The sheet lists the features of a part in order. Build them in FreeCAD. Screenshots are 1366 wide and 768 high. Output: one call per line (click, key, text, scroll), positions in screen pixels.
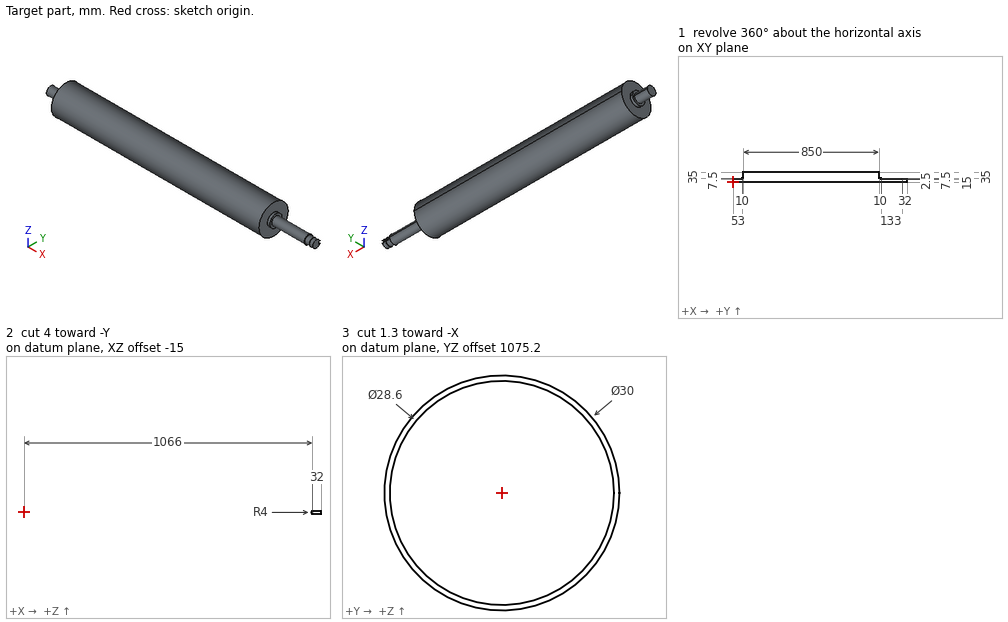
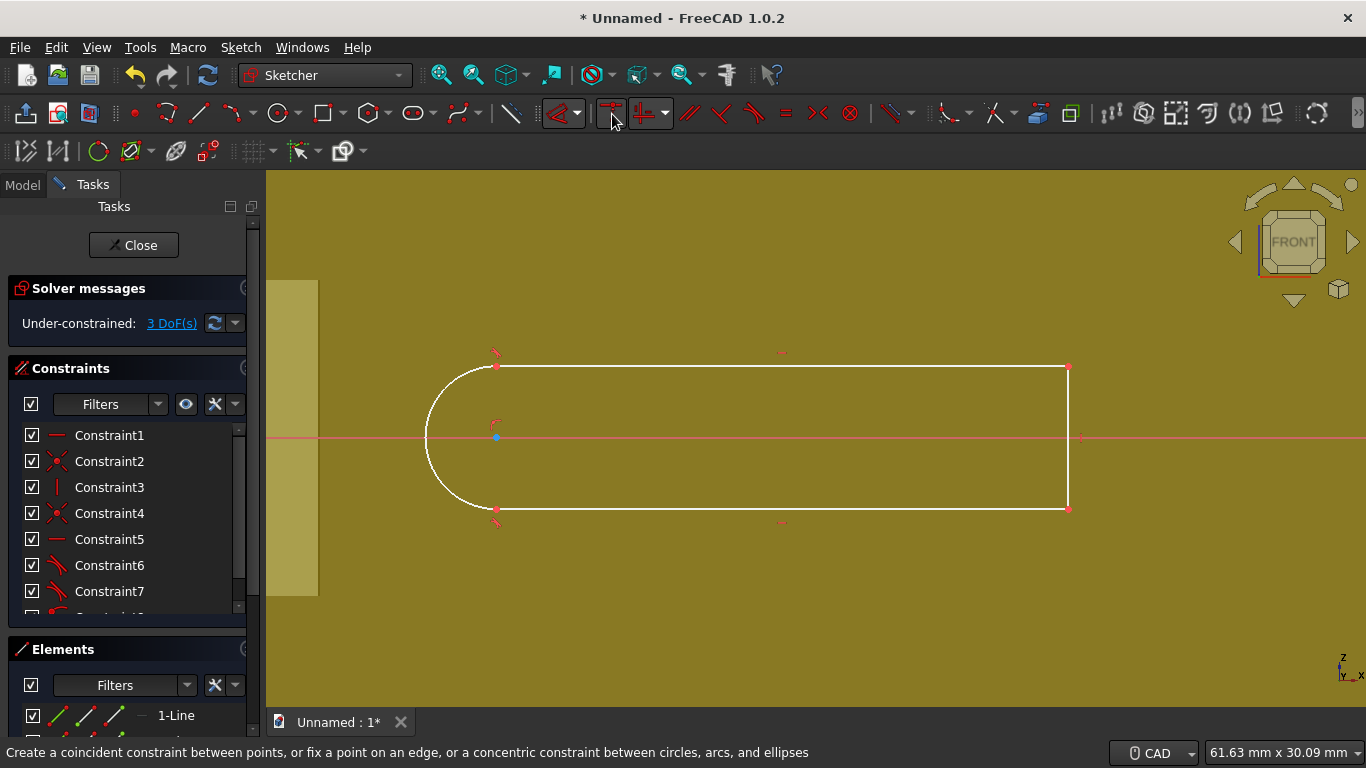
click(439, 396)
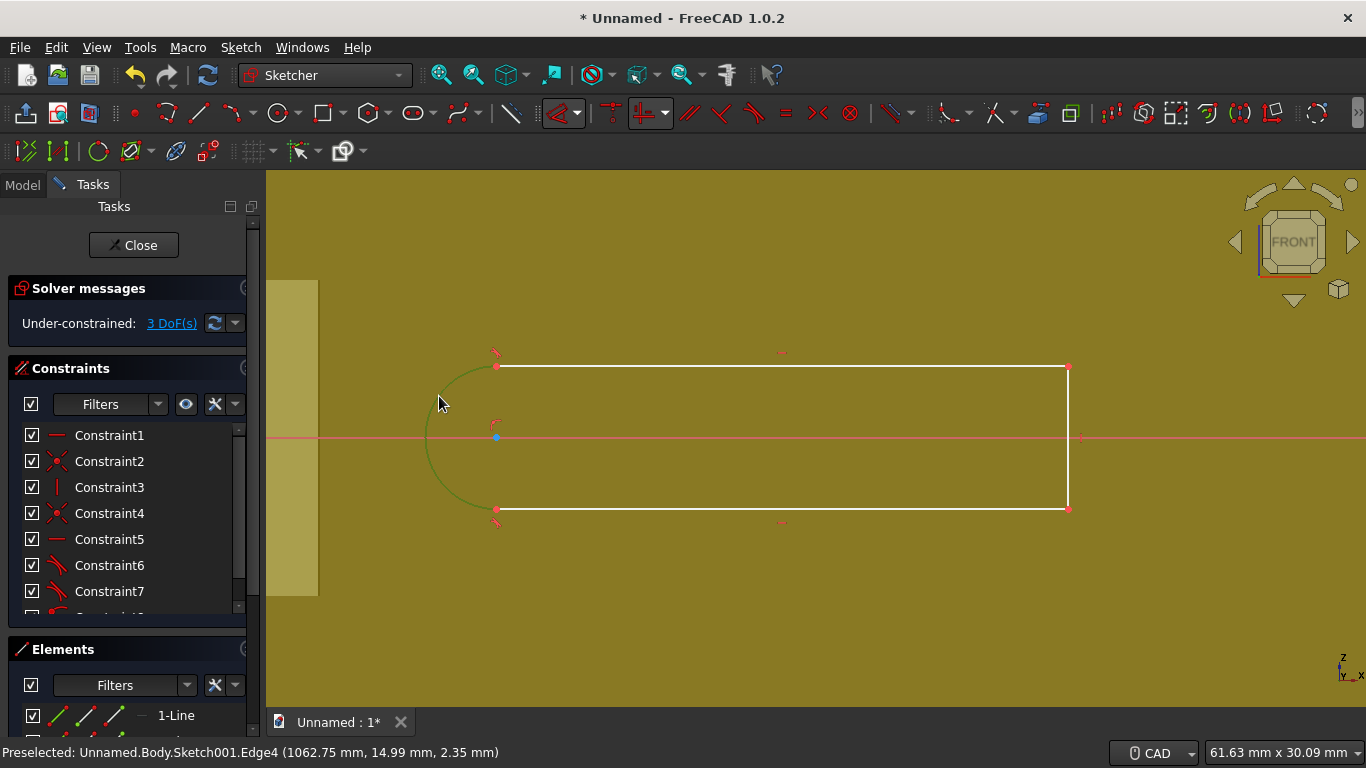
key(k)
key(r)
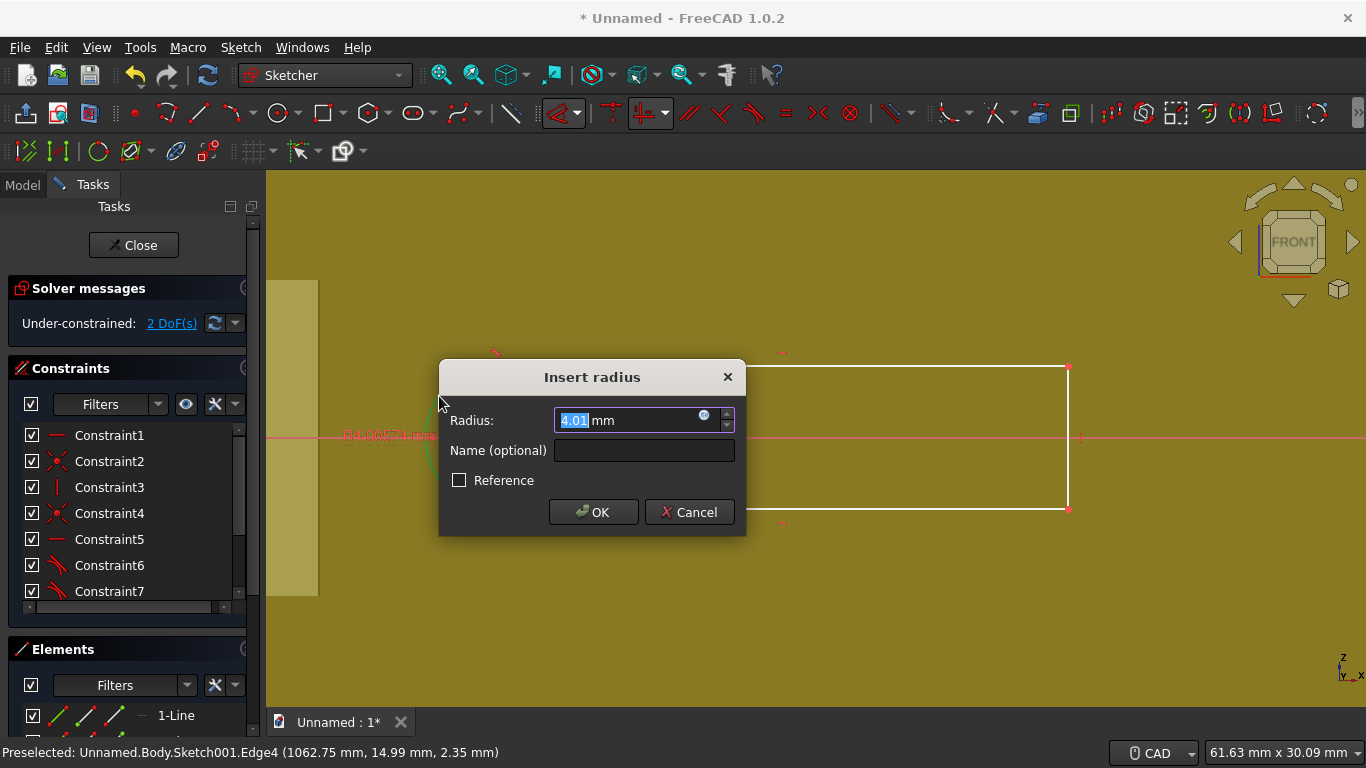
text(4)
key(Return)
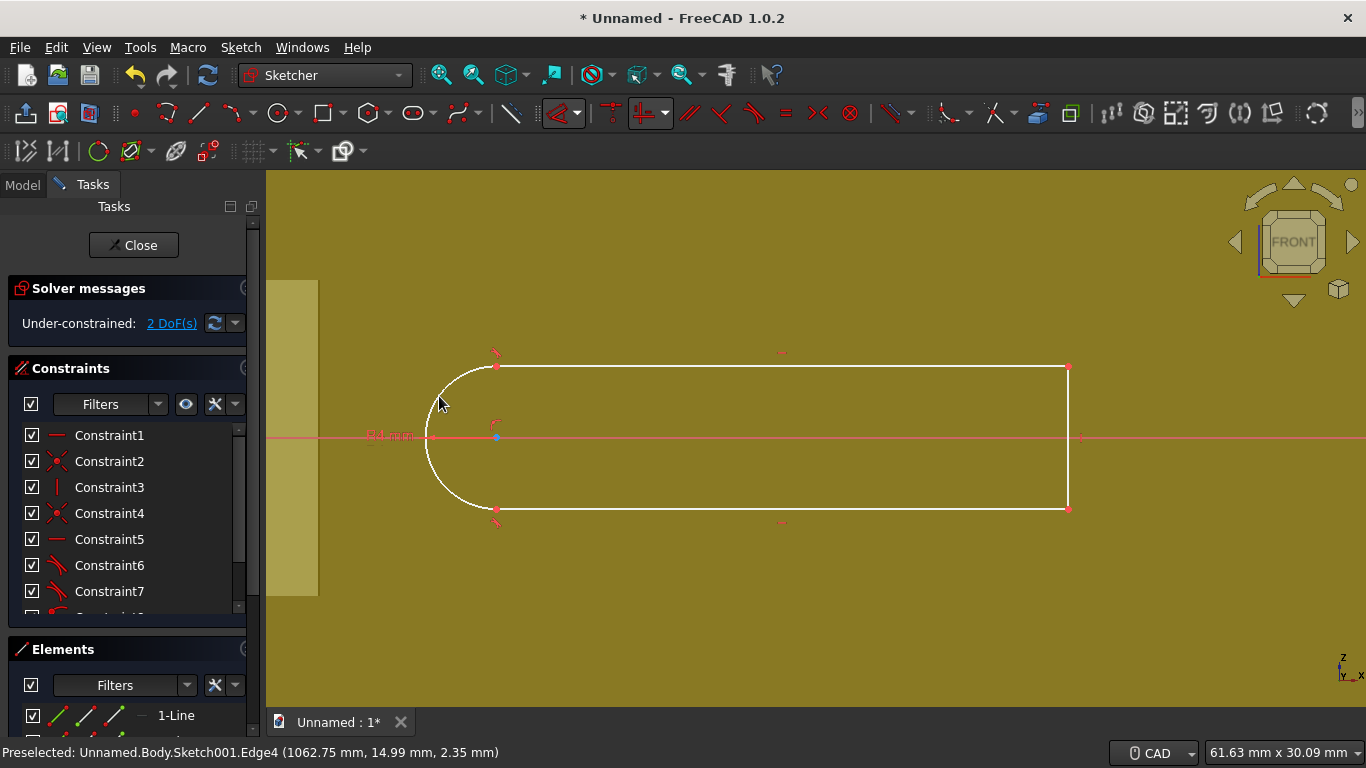
click(668, 366)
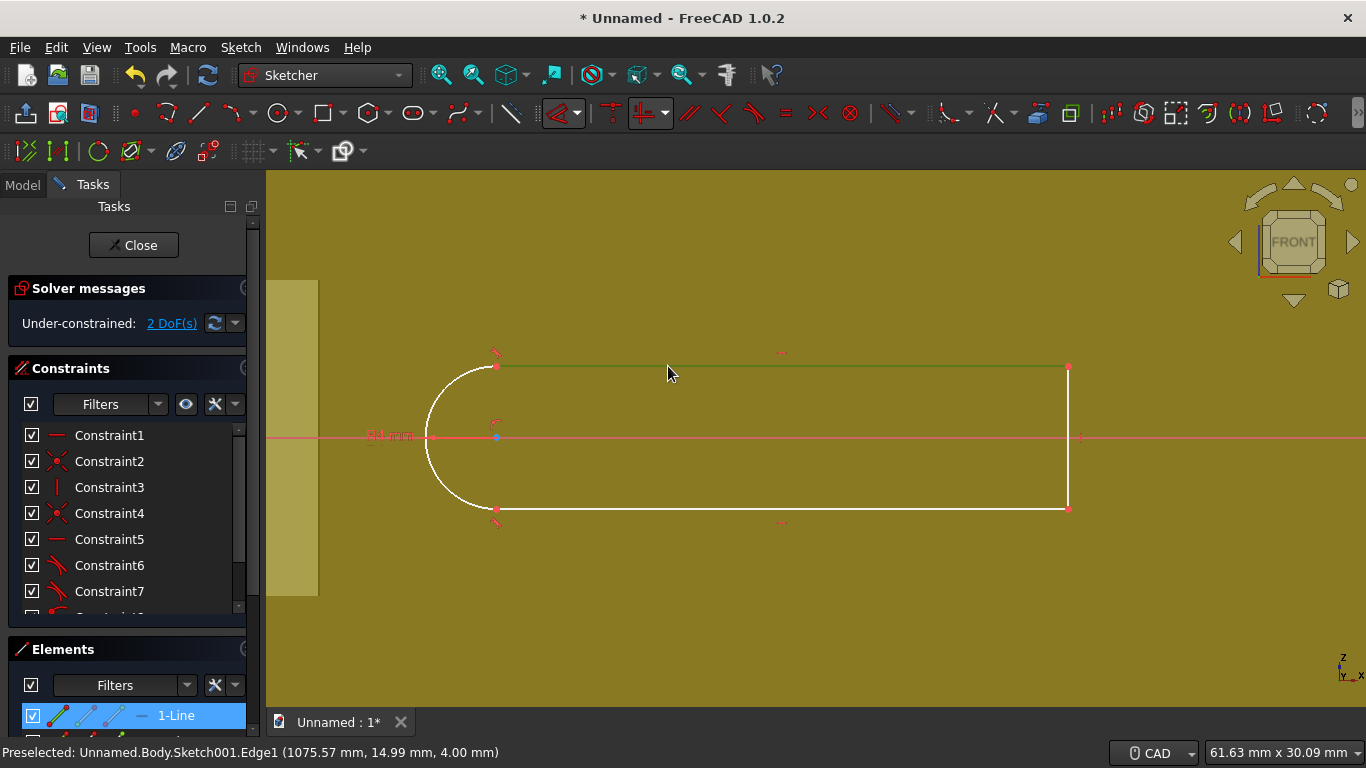
click(580, 114)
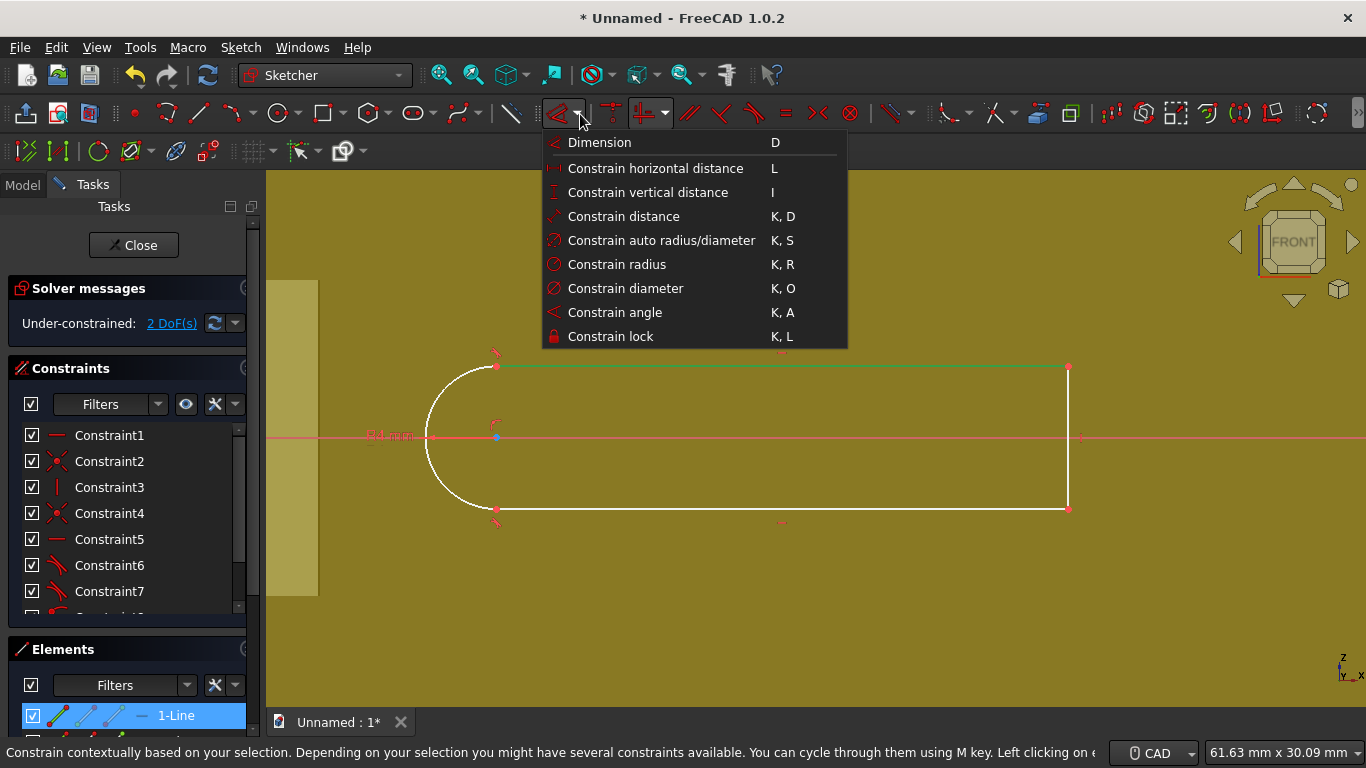
click(695, 168)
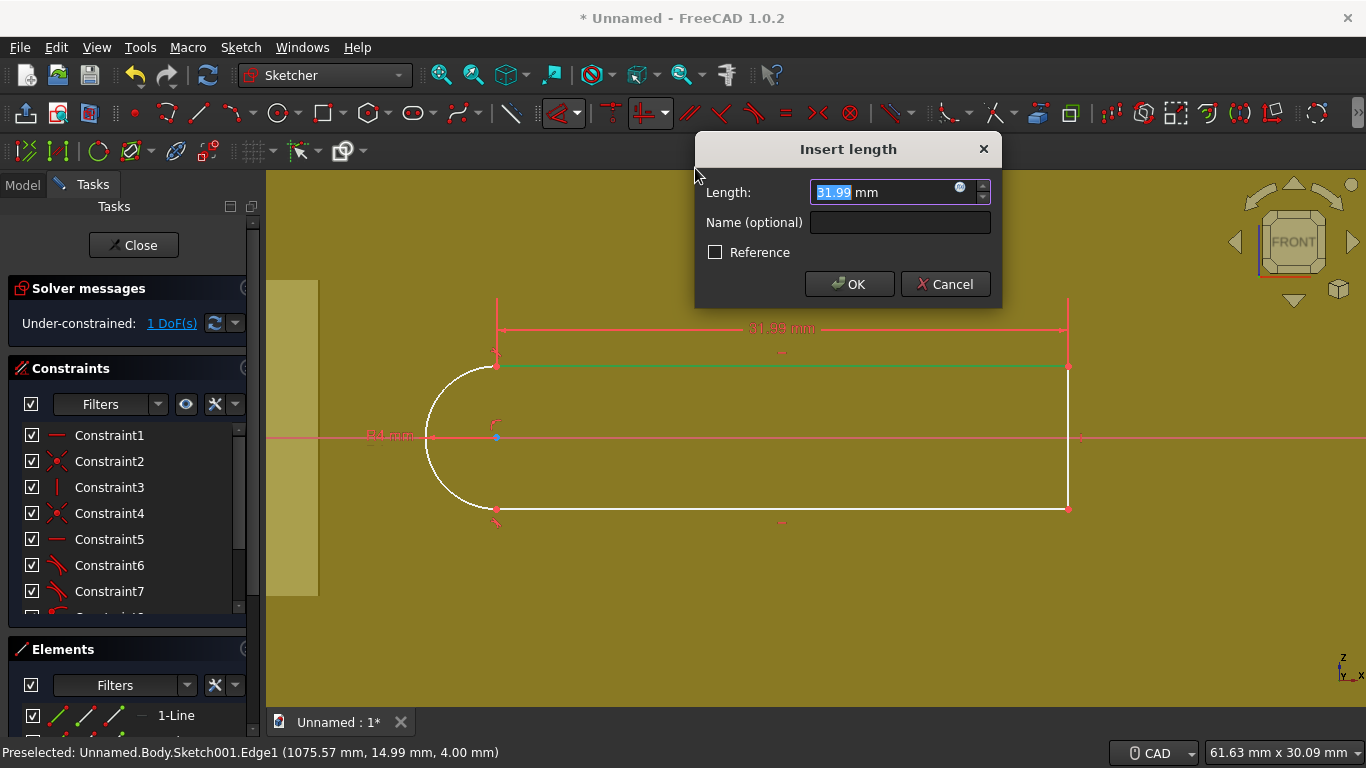
text(32)
key(Return)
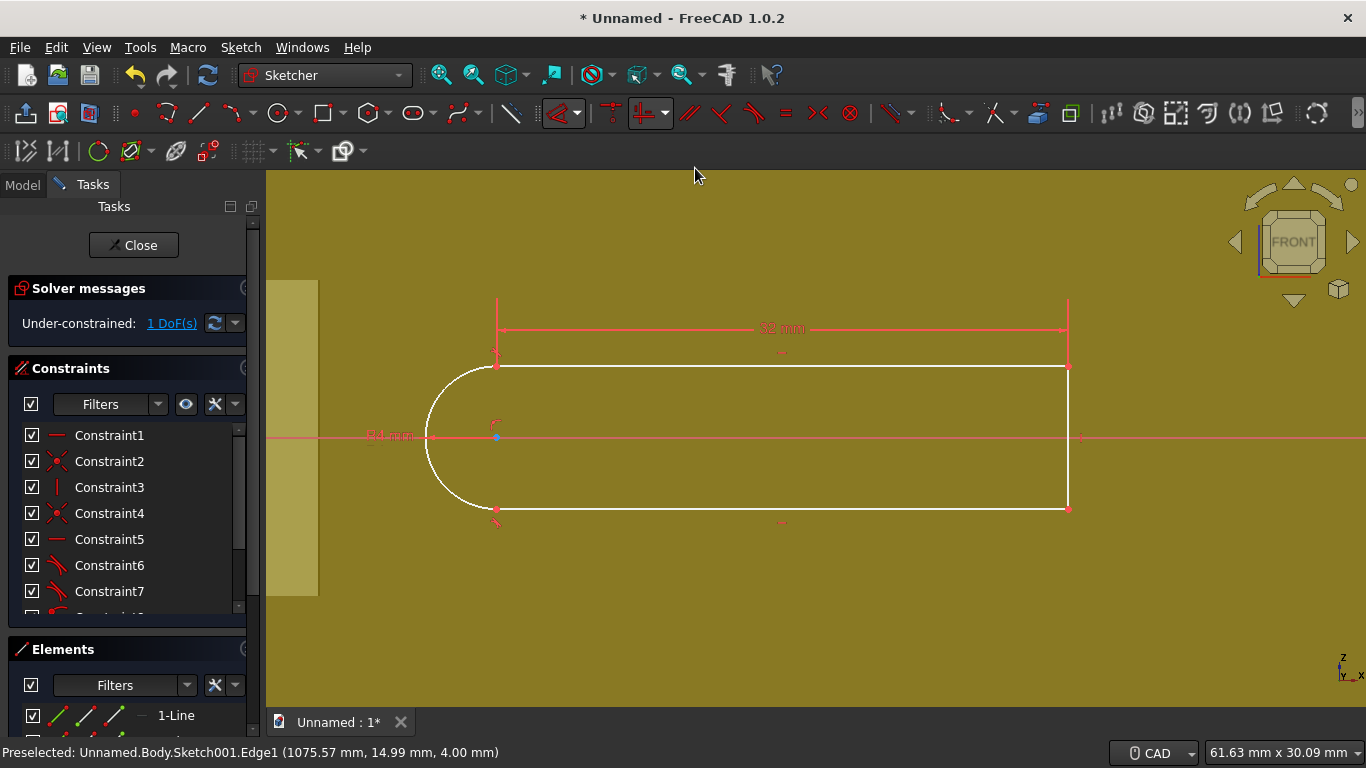
click(497, 366)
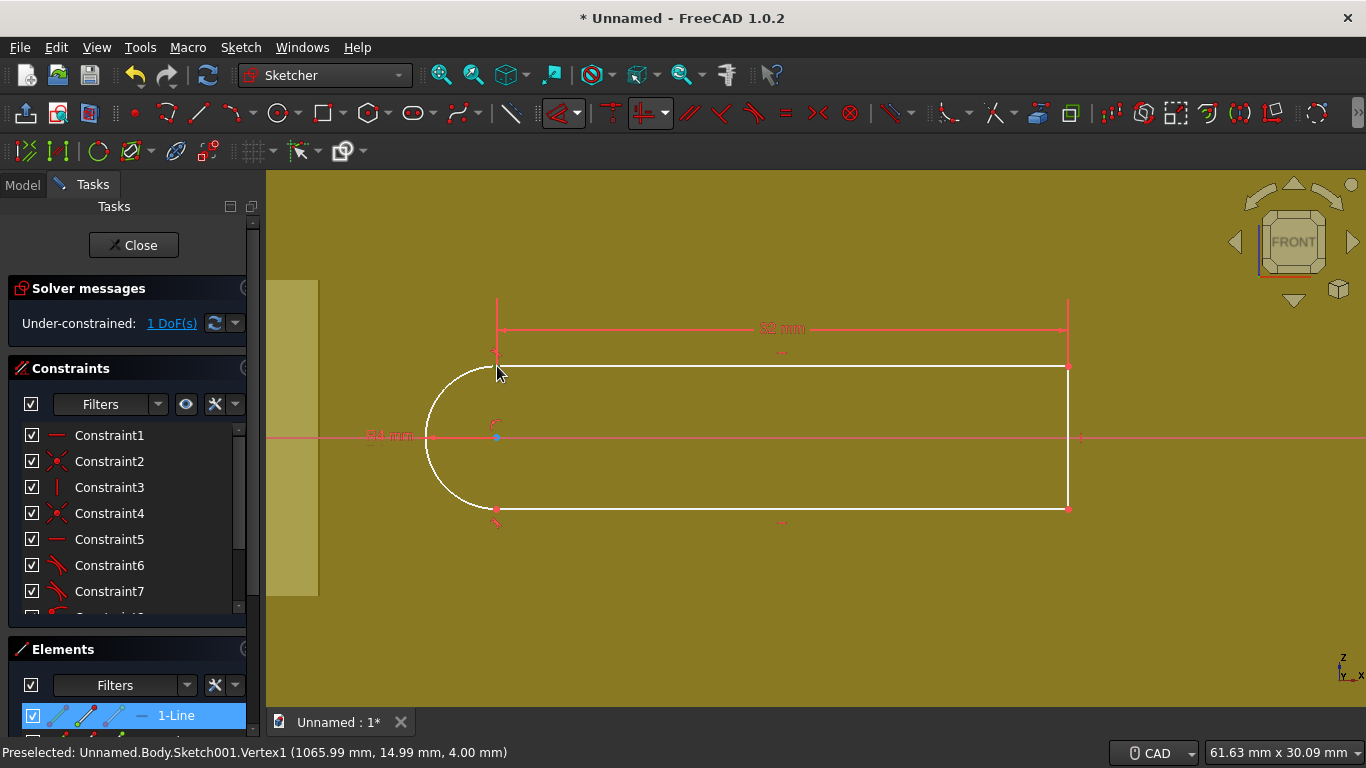
click(580, 114)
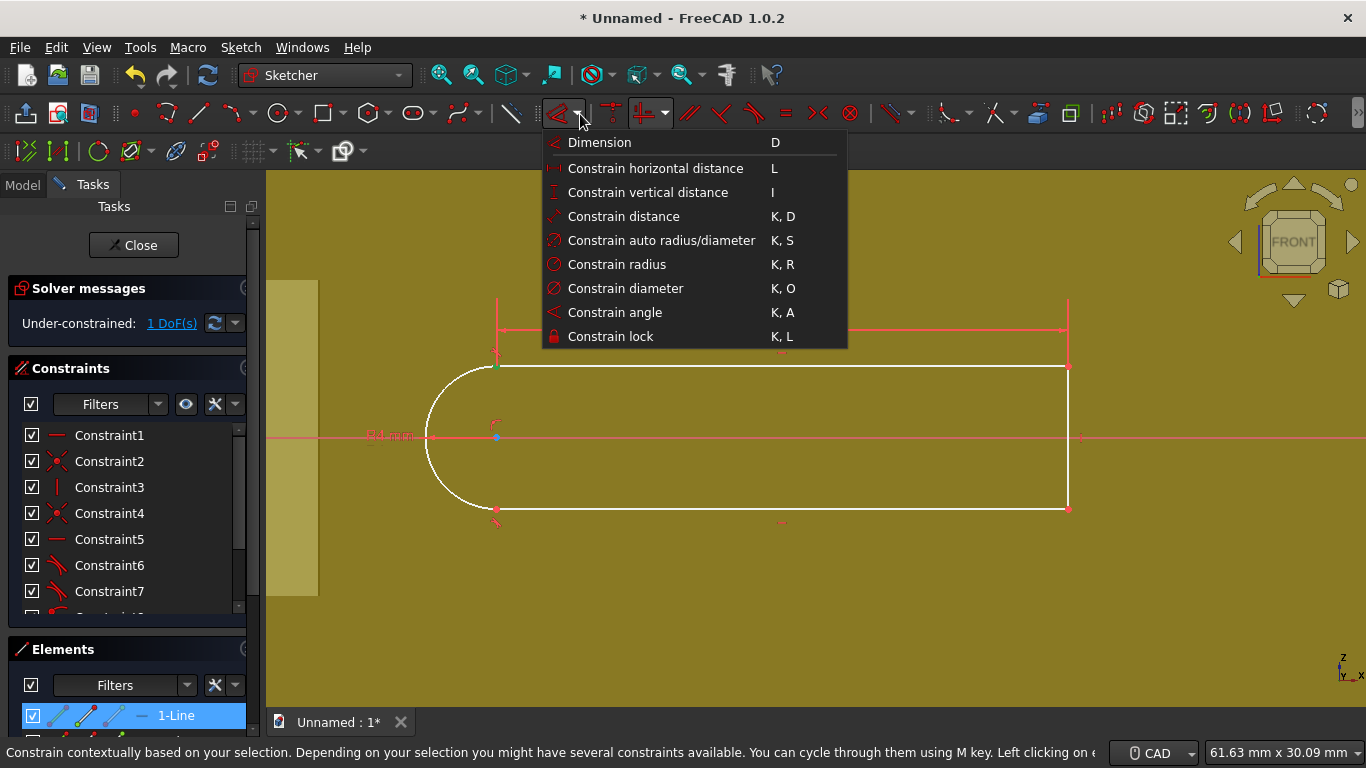
click(695, 168)